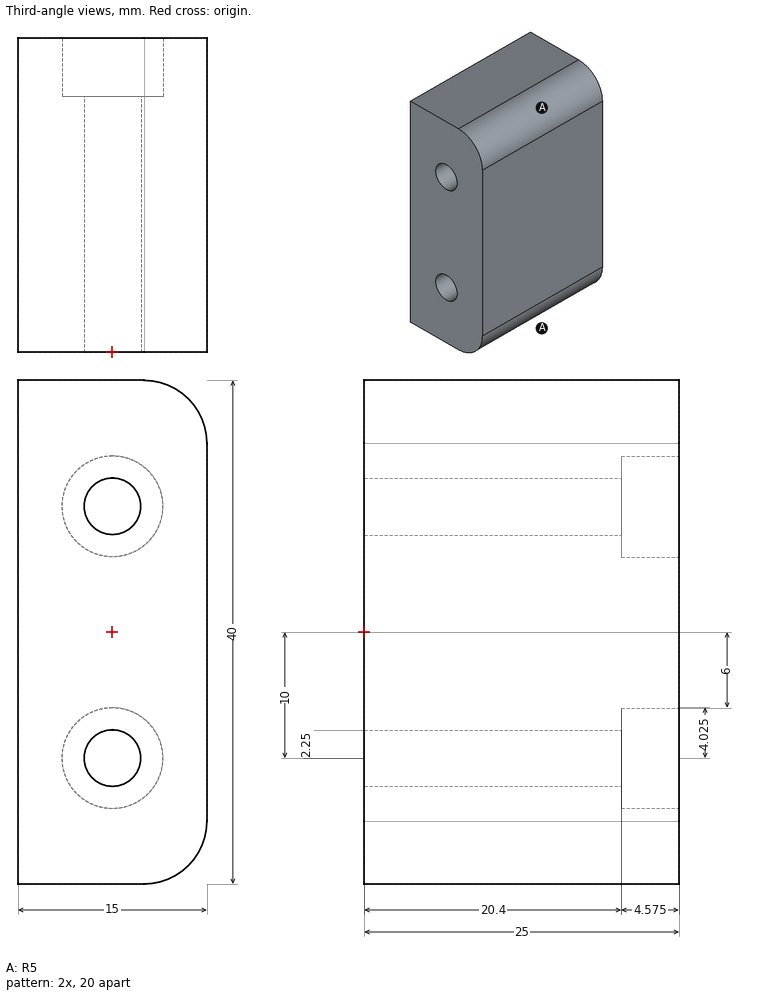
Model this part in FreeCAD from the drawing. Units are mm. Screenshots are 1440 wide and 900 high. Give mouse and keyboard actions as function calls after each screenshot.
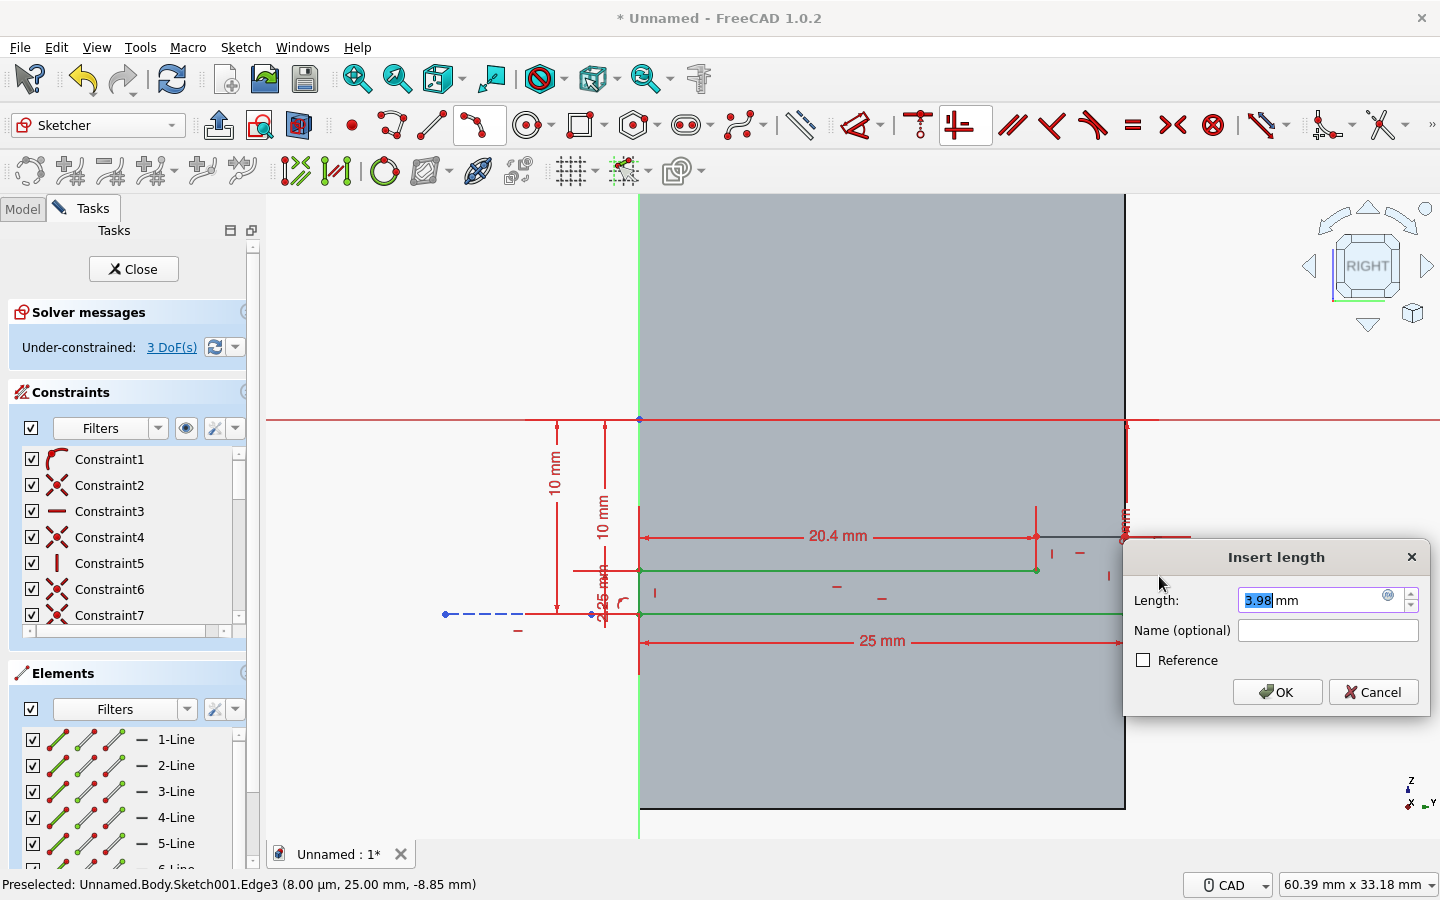
text(4.025)
key(Return)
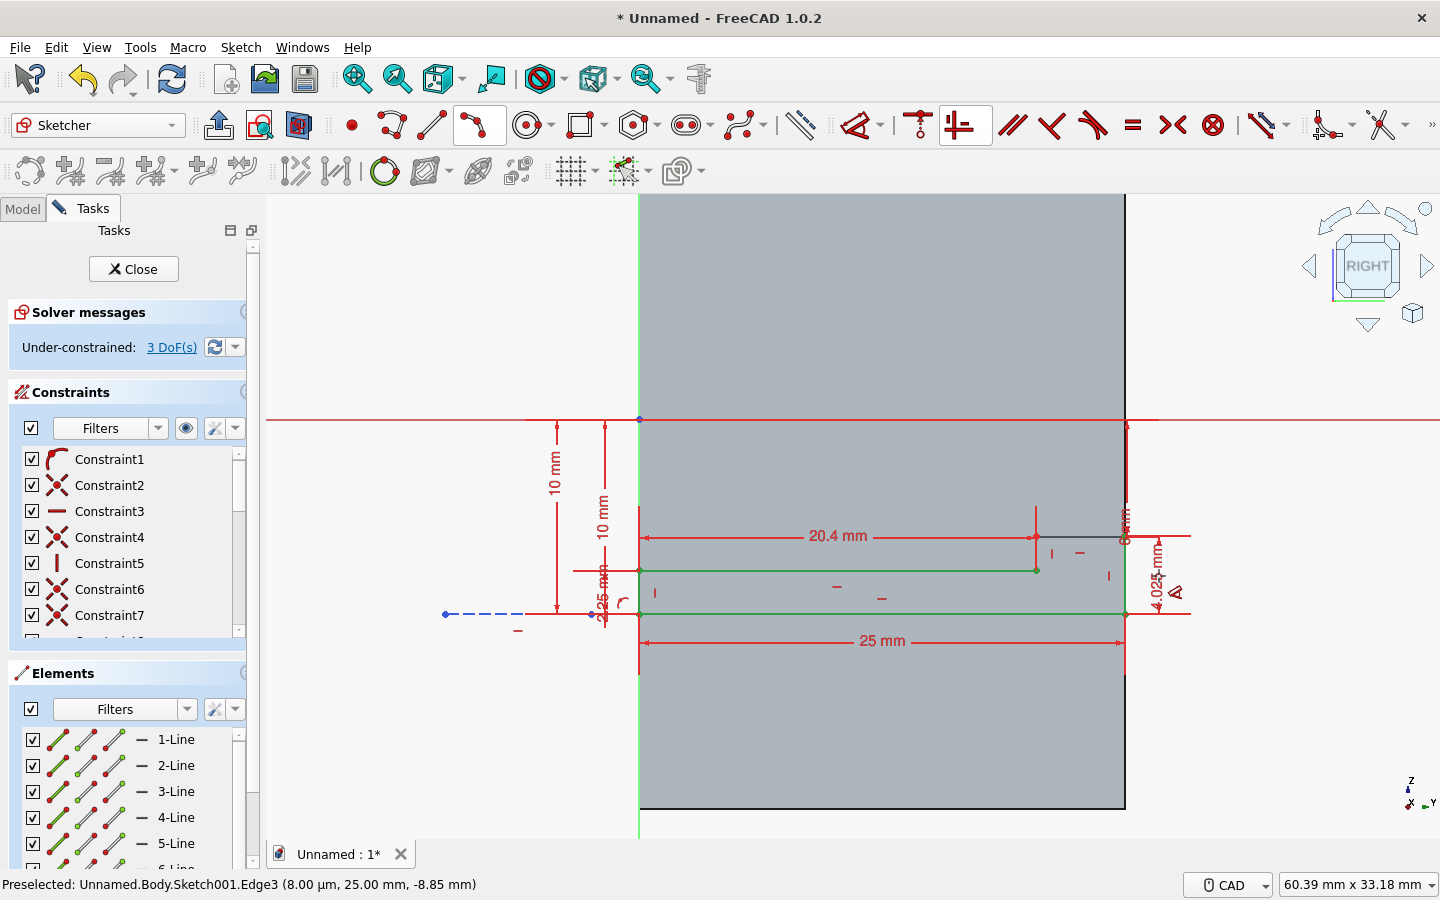
click(1098, 537)
click(1081, 571)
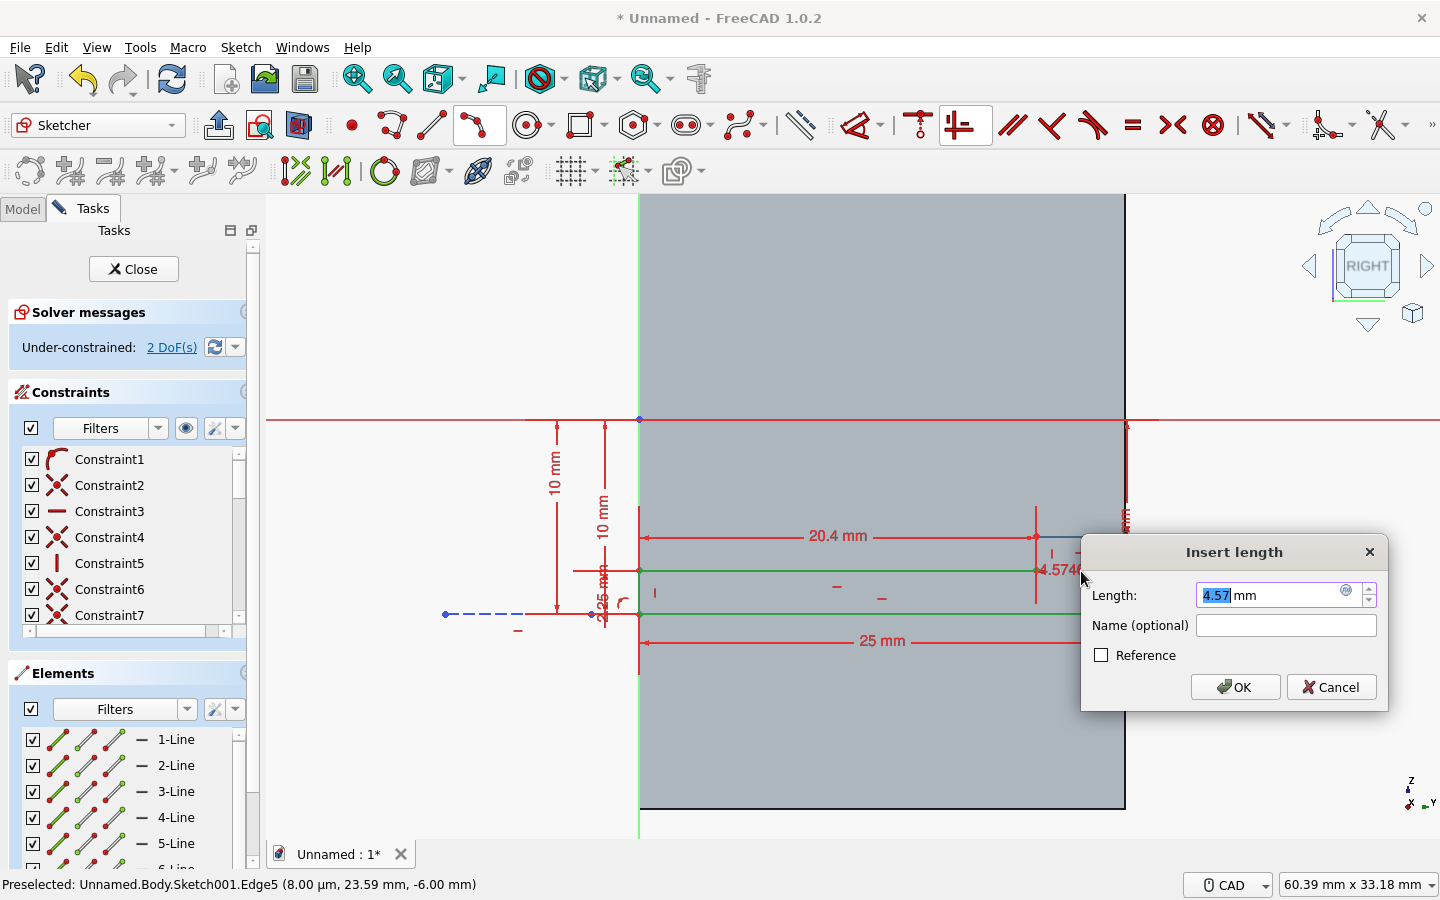
text(4.575)
key(Return)
key(Escape)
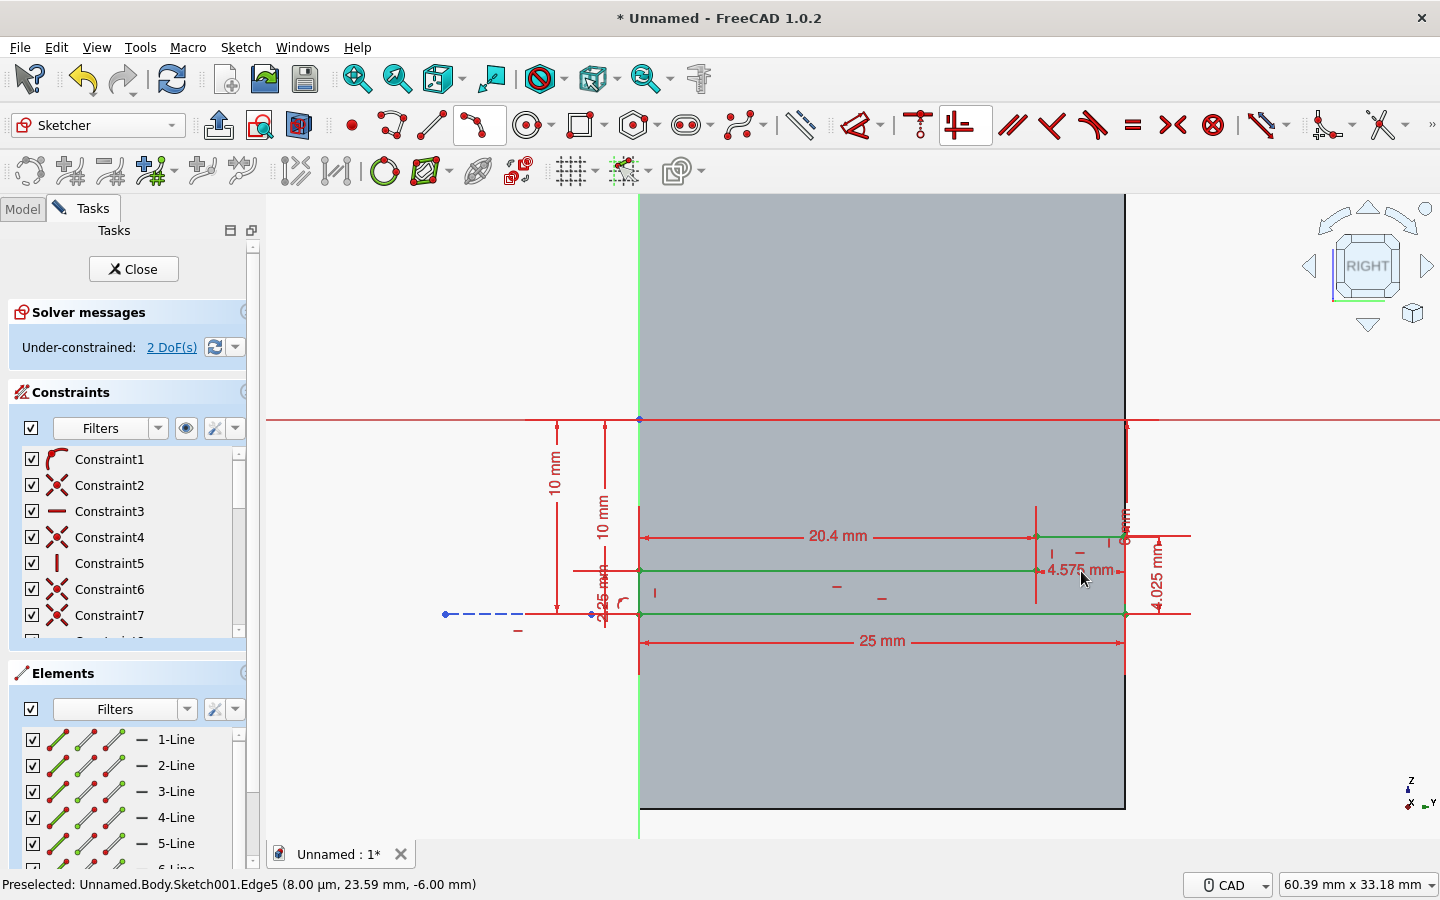
click(134, 269)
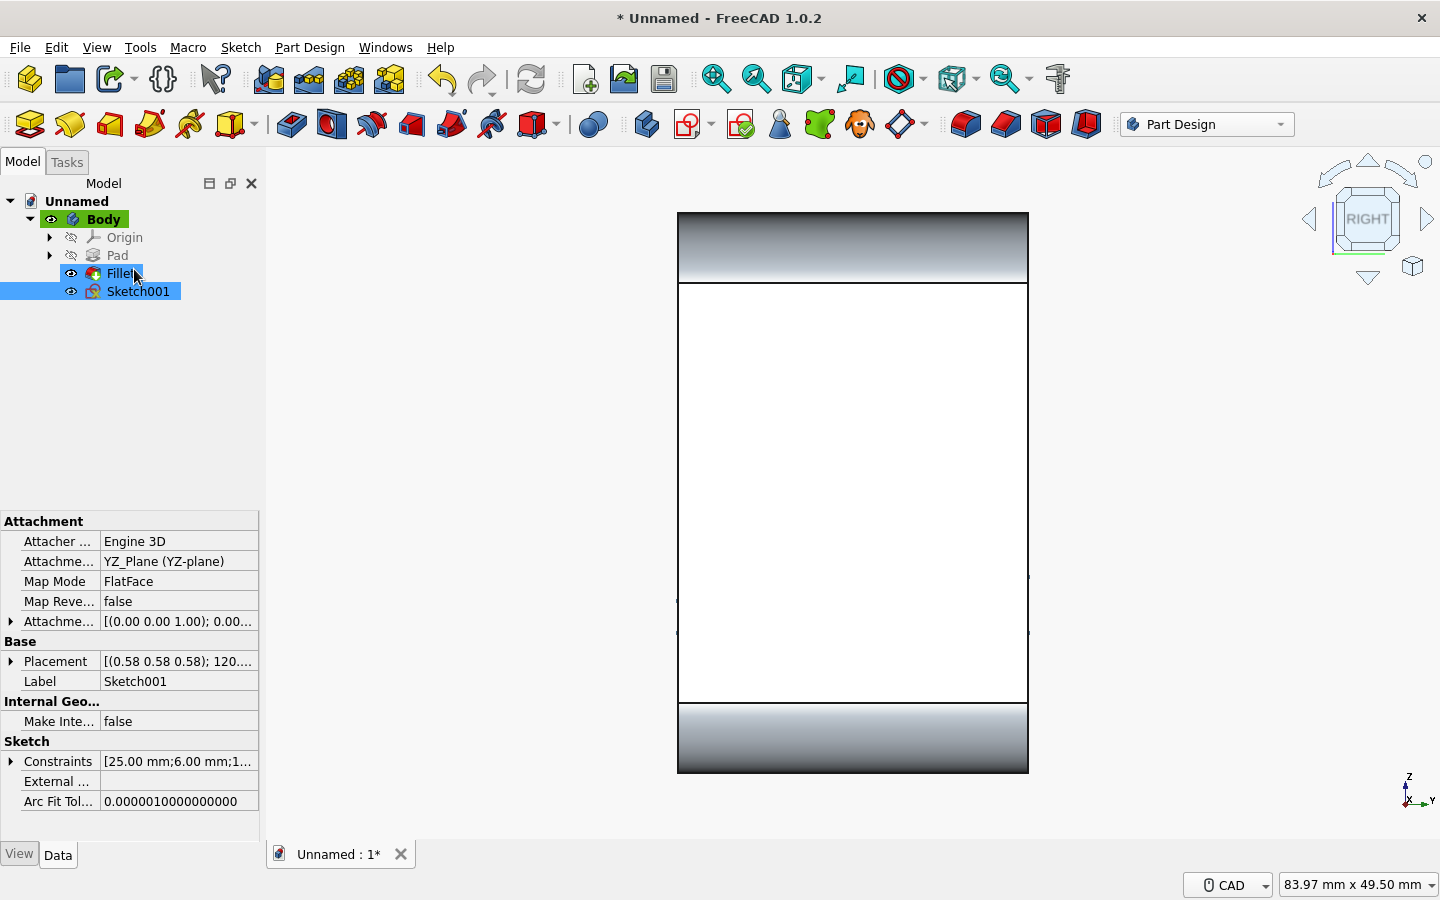
click(372, 124)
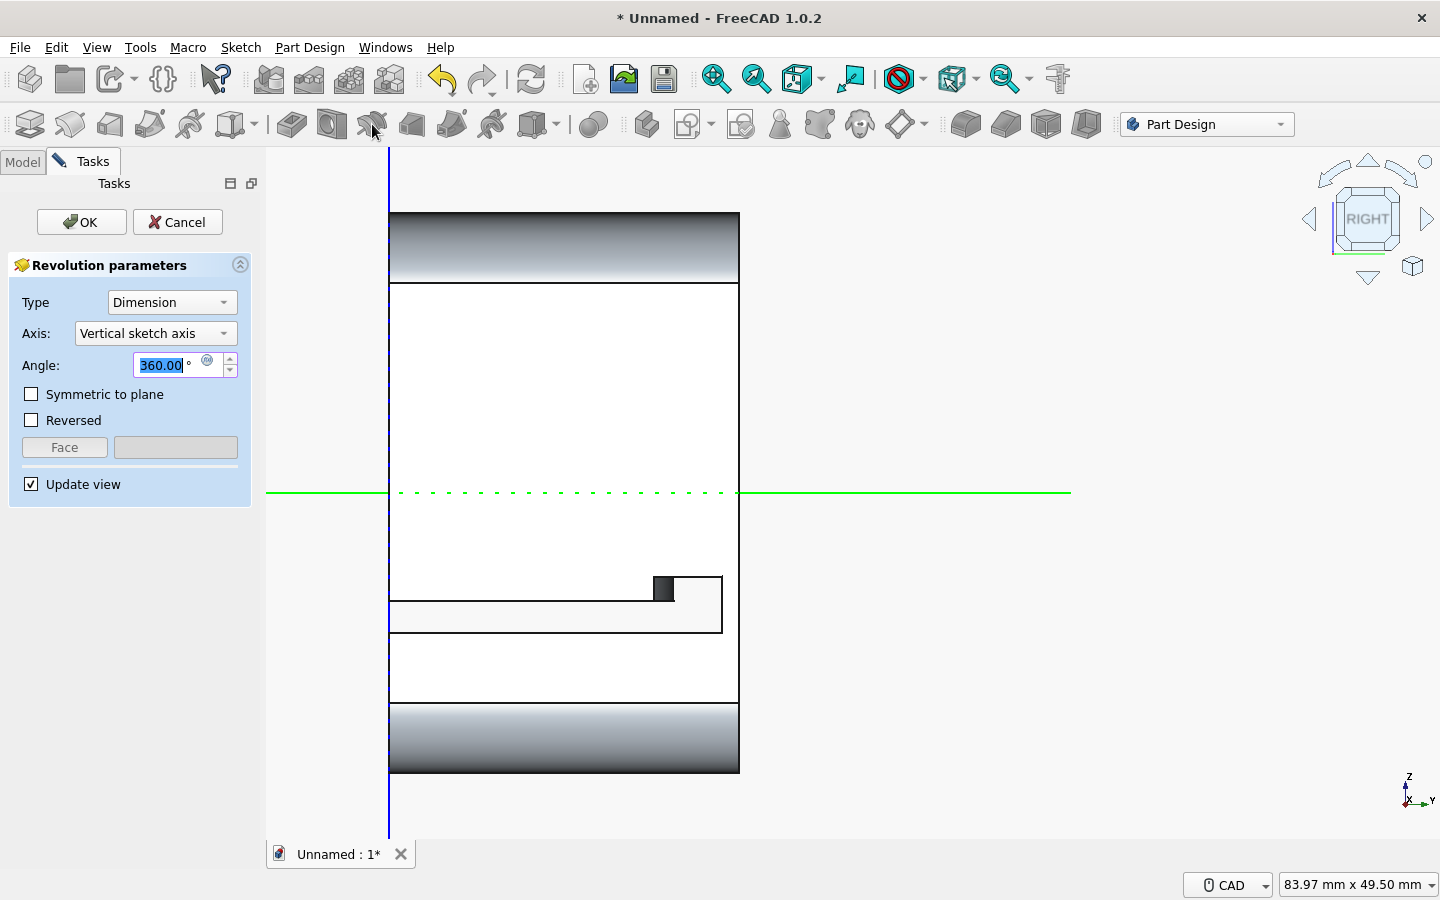
click(156, 334)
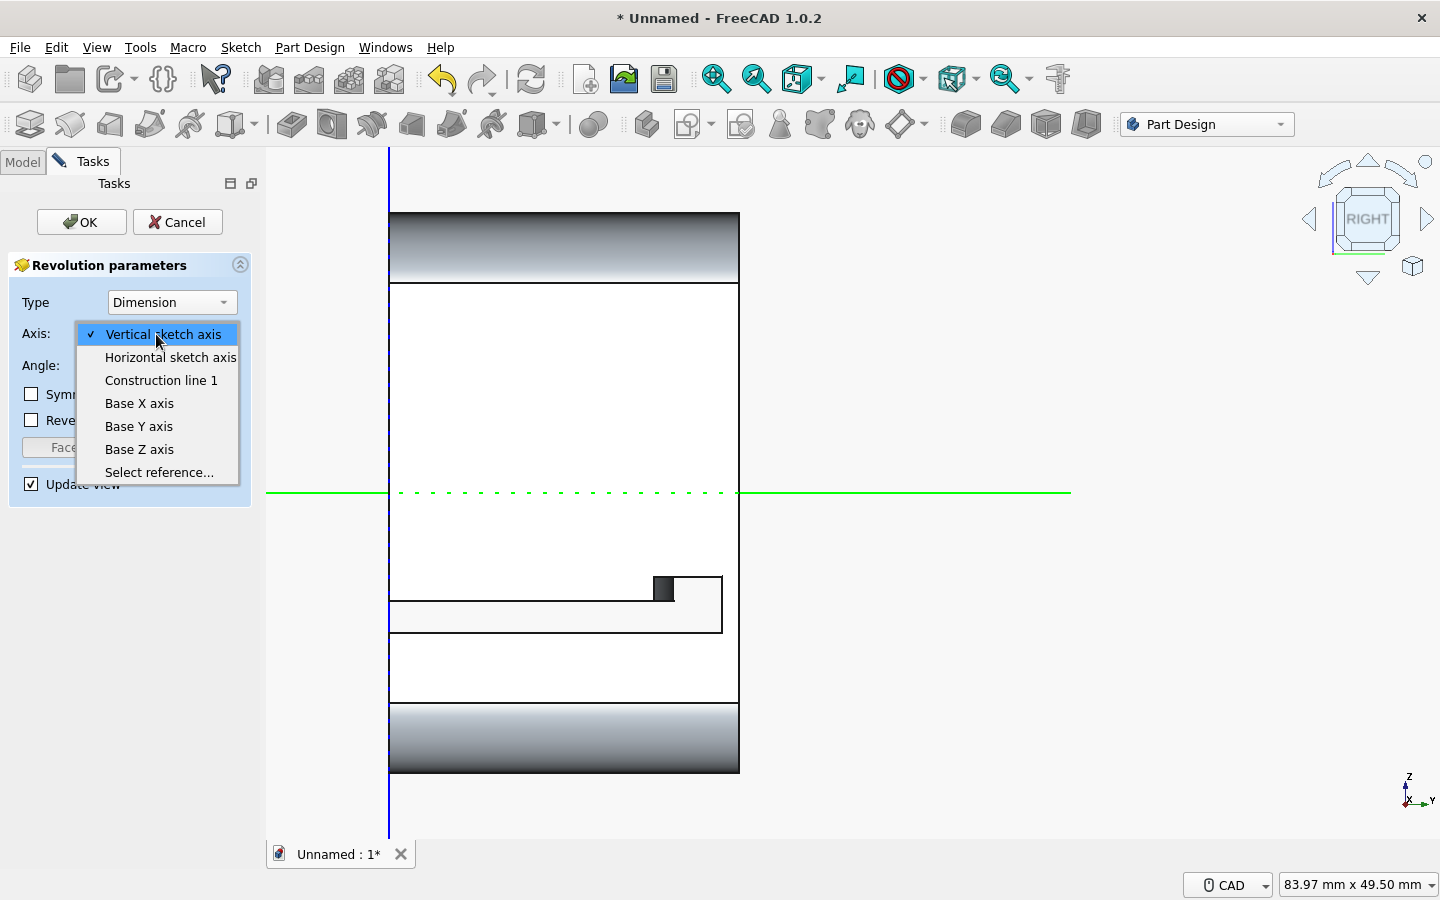
click(156, 380)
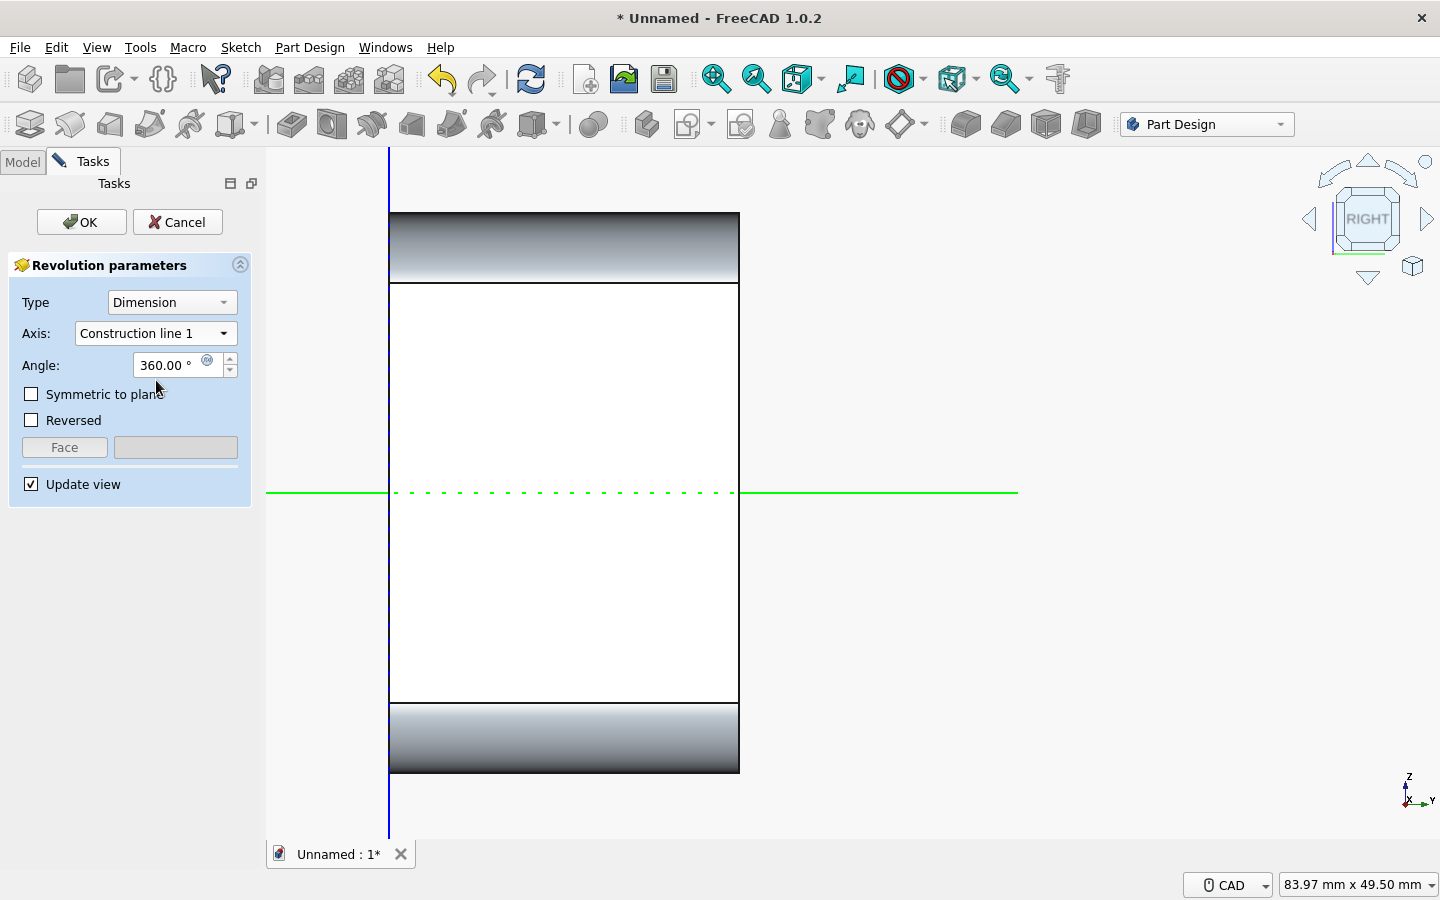
click(82, 222)